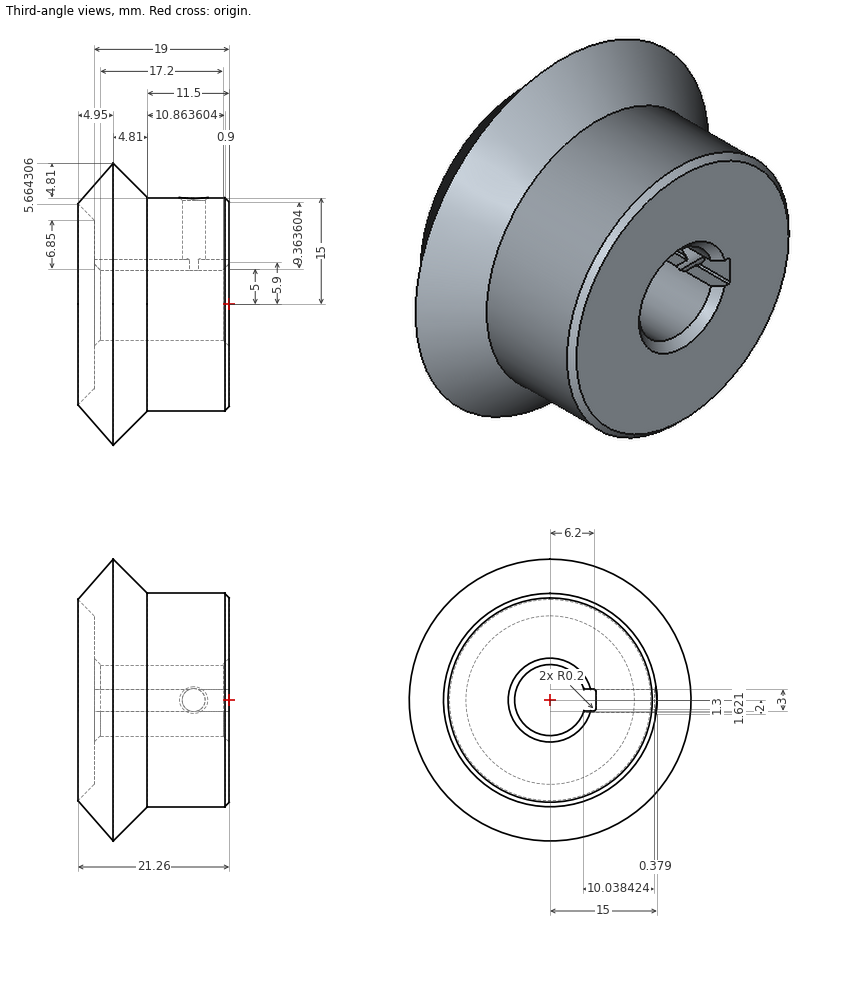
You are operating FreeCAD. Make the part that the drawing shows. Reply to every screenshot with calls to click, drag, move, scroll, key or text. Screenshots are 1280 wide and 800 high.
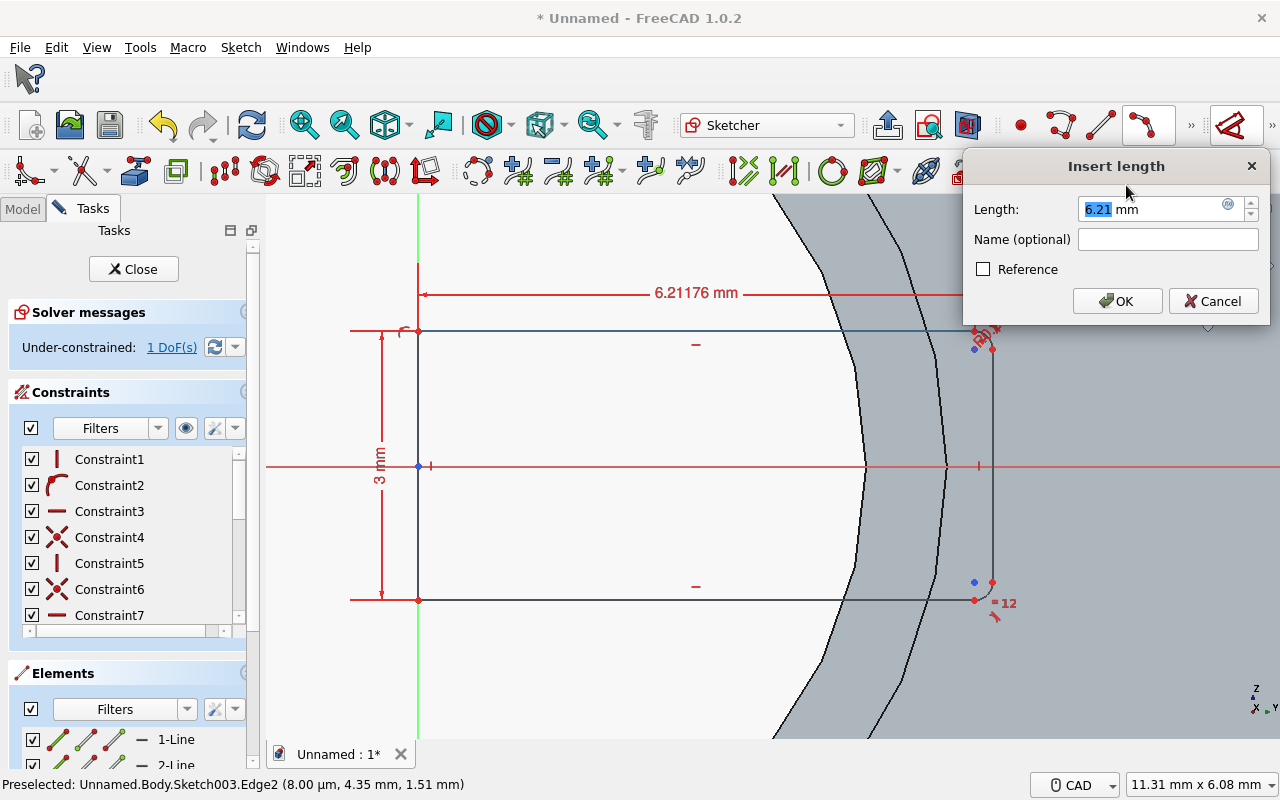
text(6.2)
key(Return)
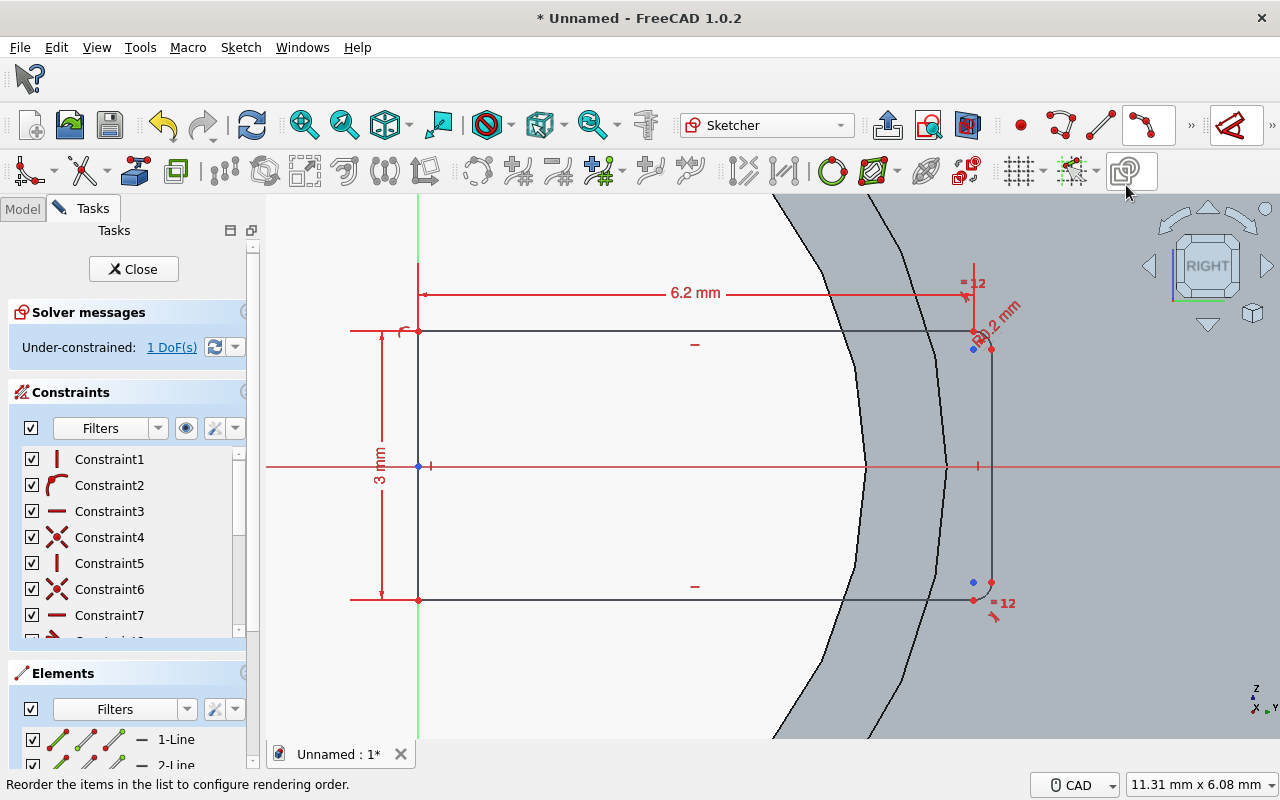
click(992, 582)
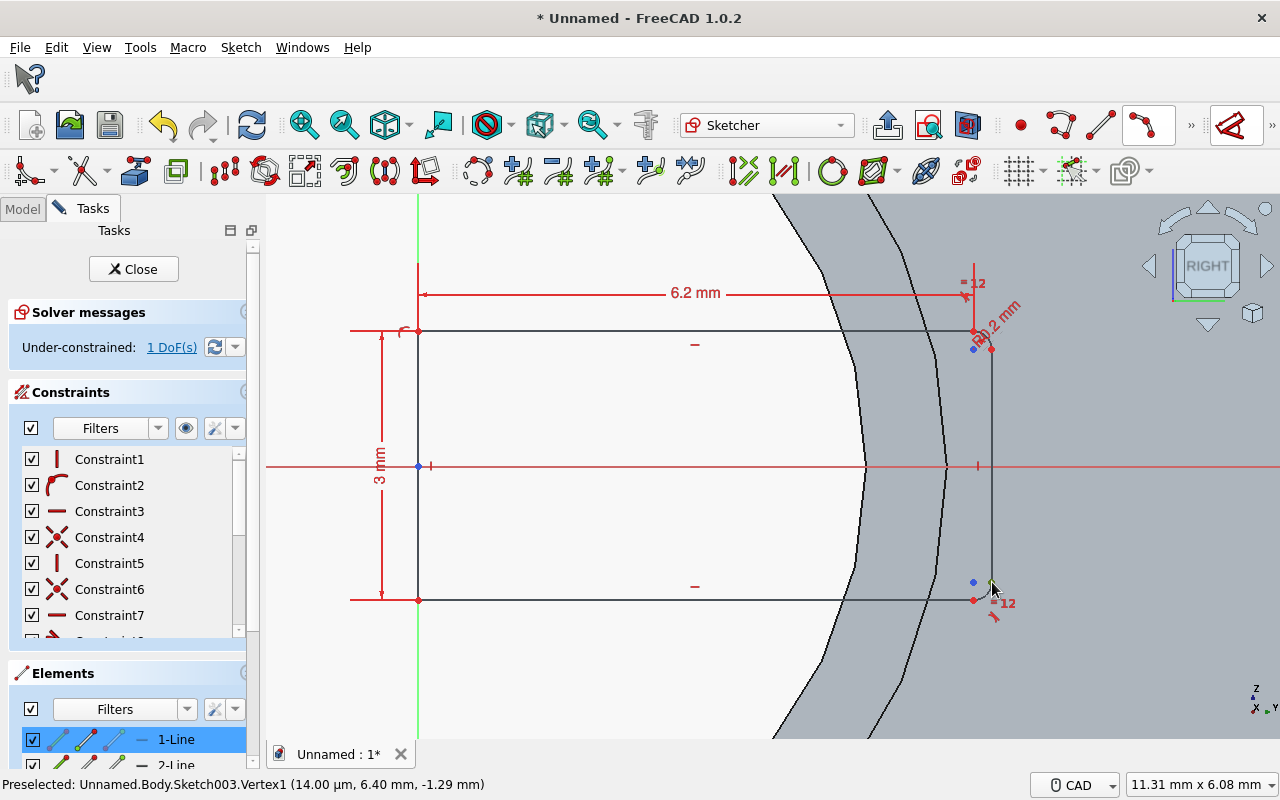
key(i)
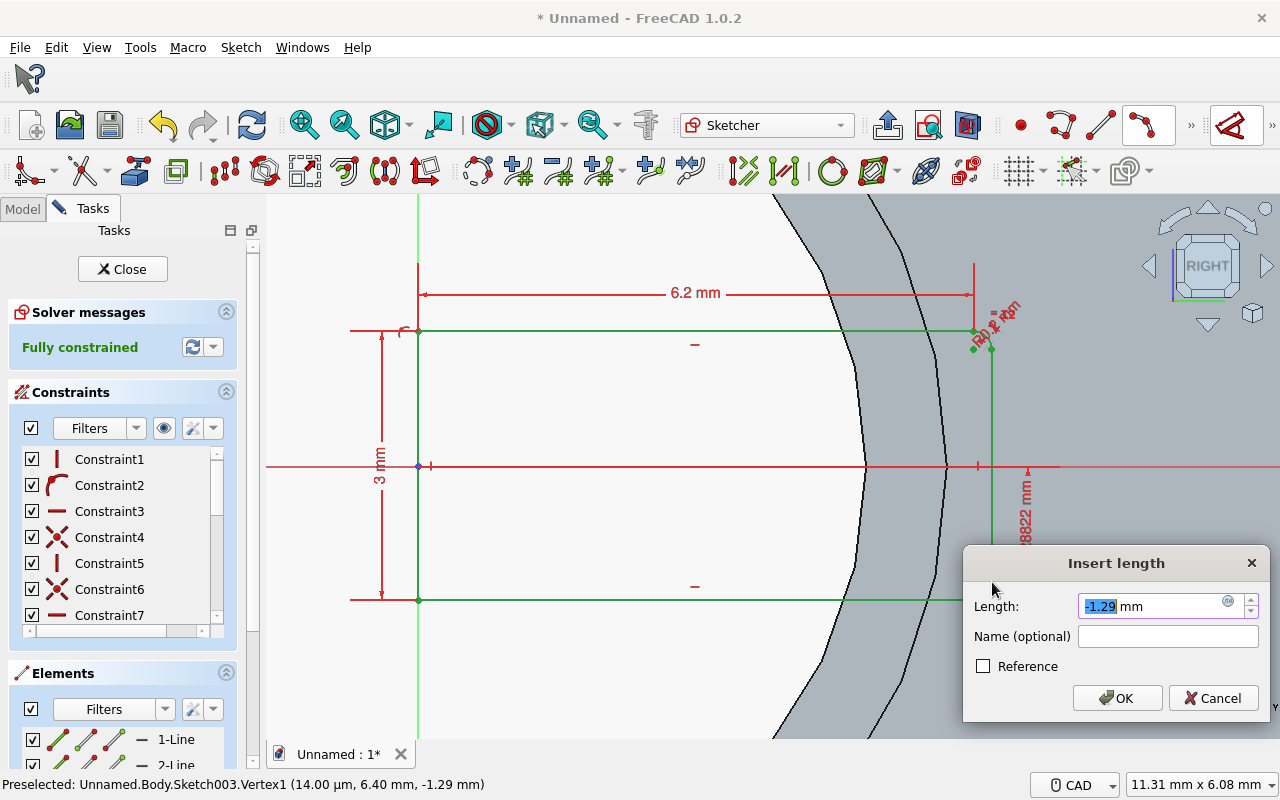
text(-1.3)
key(Return)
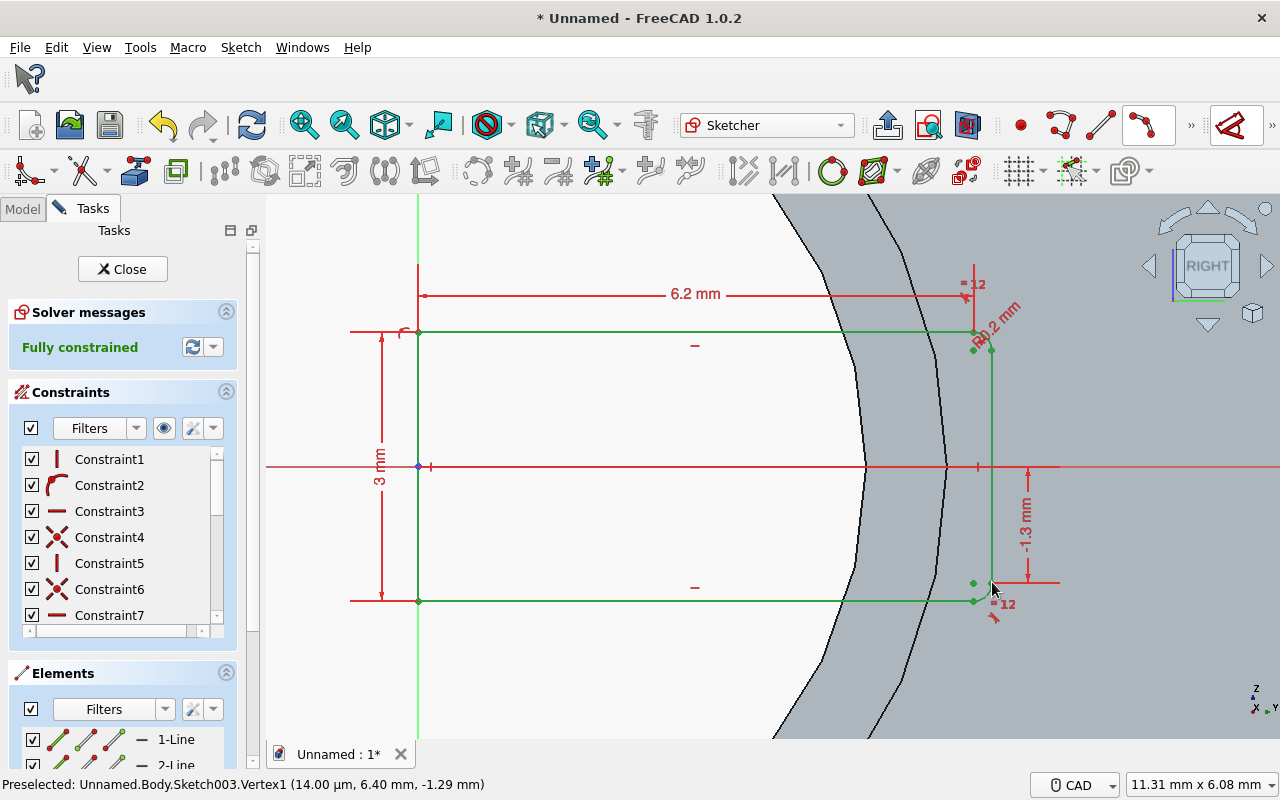
click(123, 269)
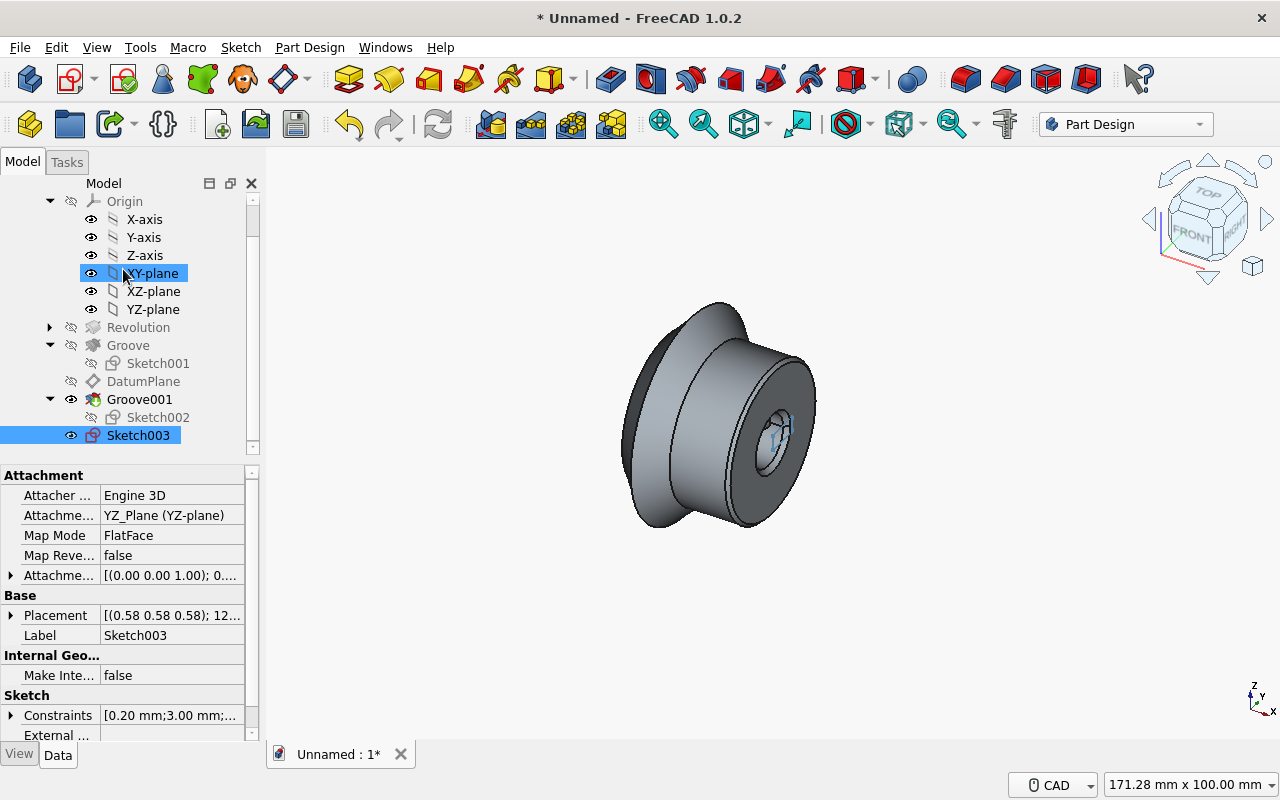
click(612, 80)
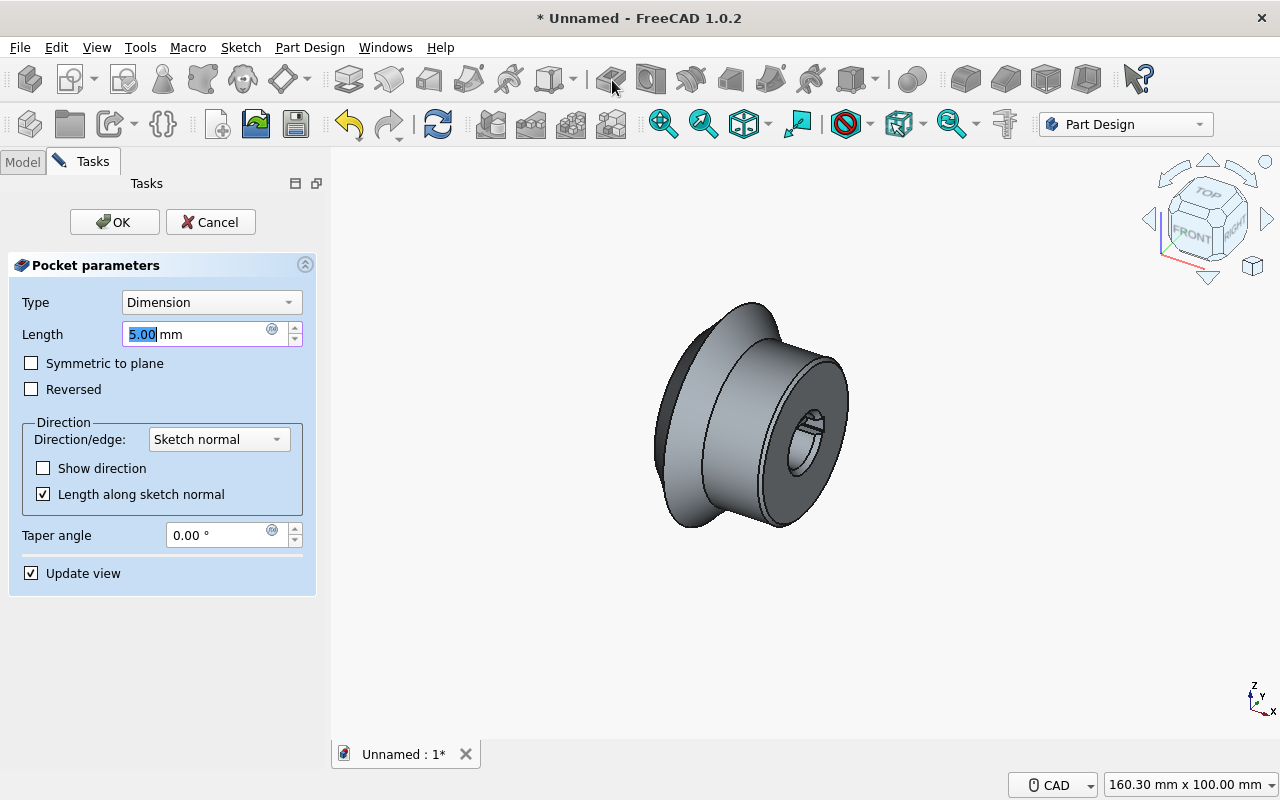
text(21.26)
key(Tab)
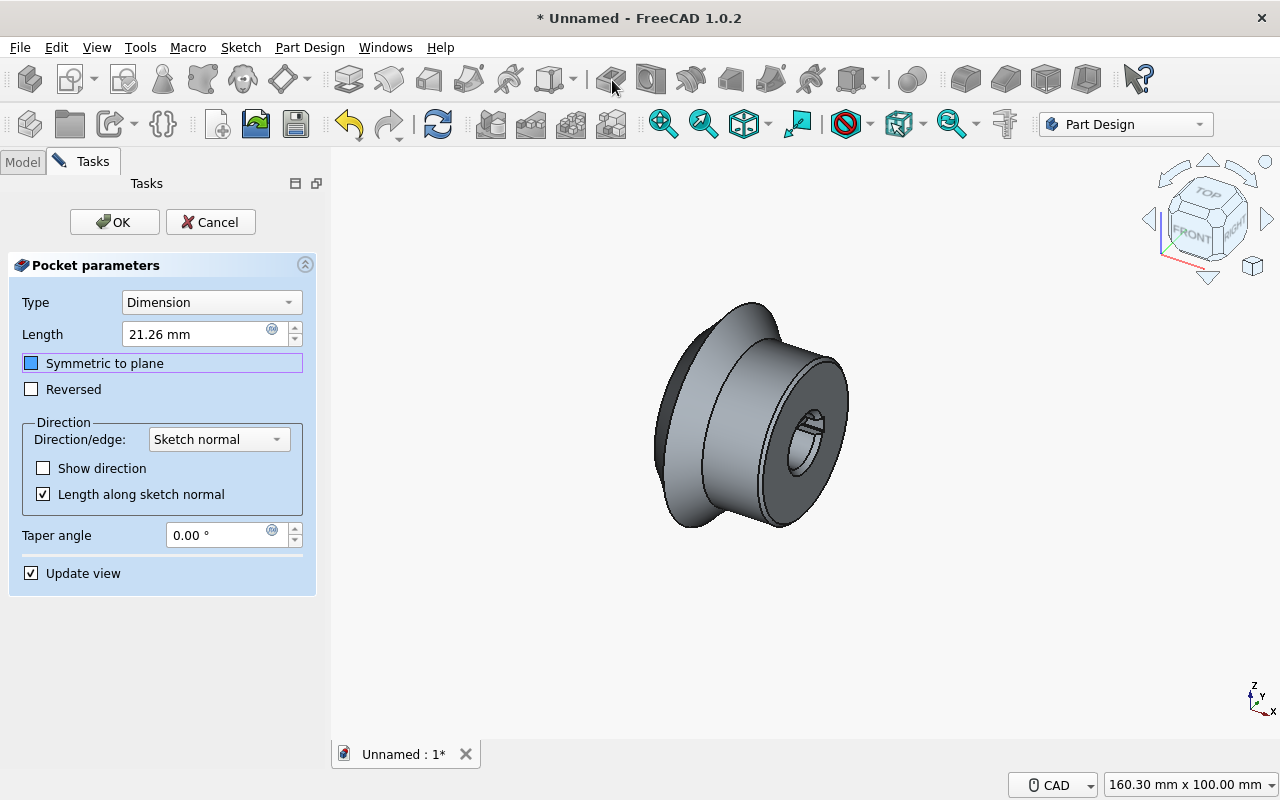
click(115, 222)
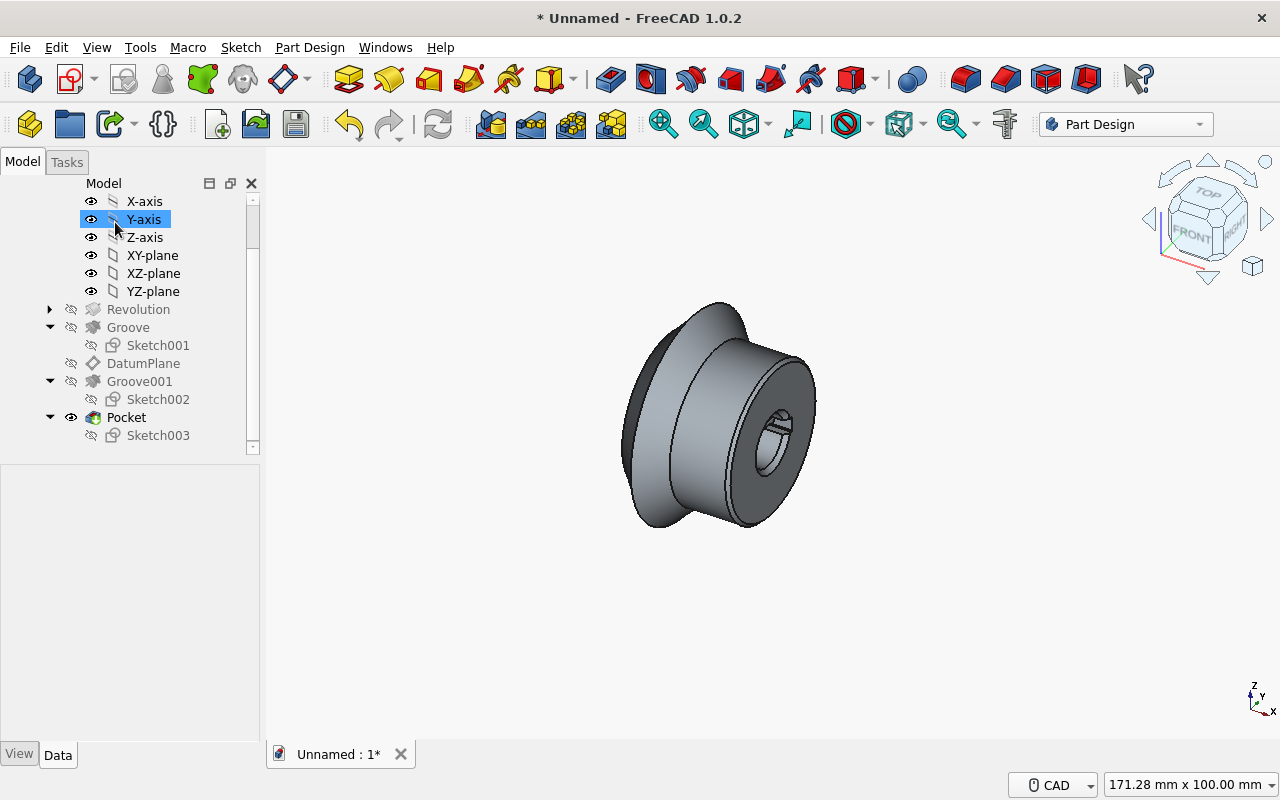
key(0)